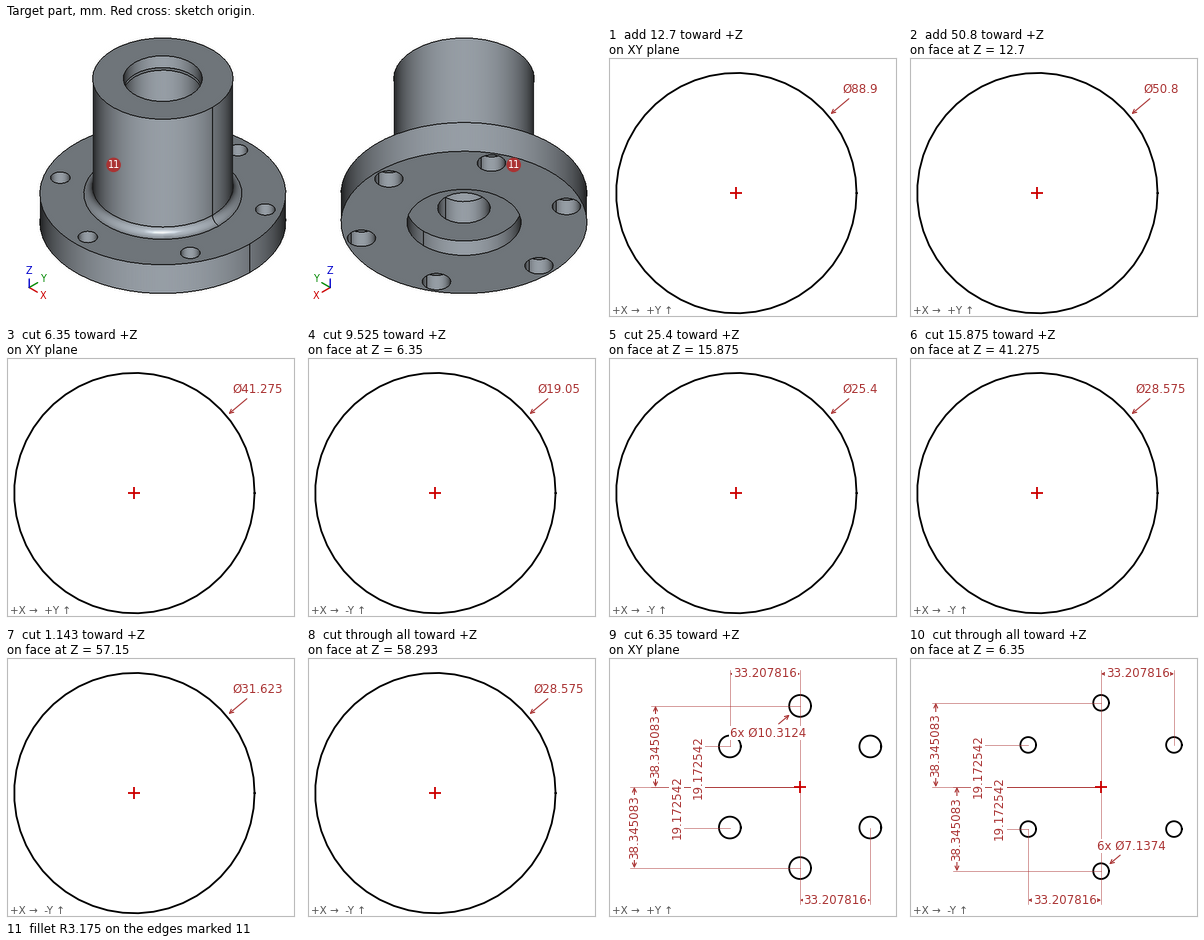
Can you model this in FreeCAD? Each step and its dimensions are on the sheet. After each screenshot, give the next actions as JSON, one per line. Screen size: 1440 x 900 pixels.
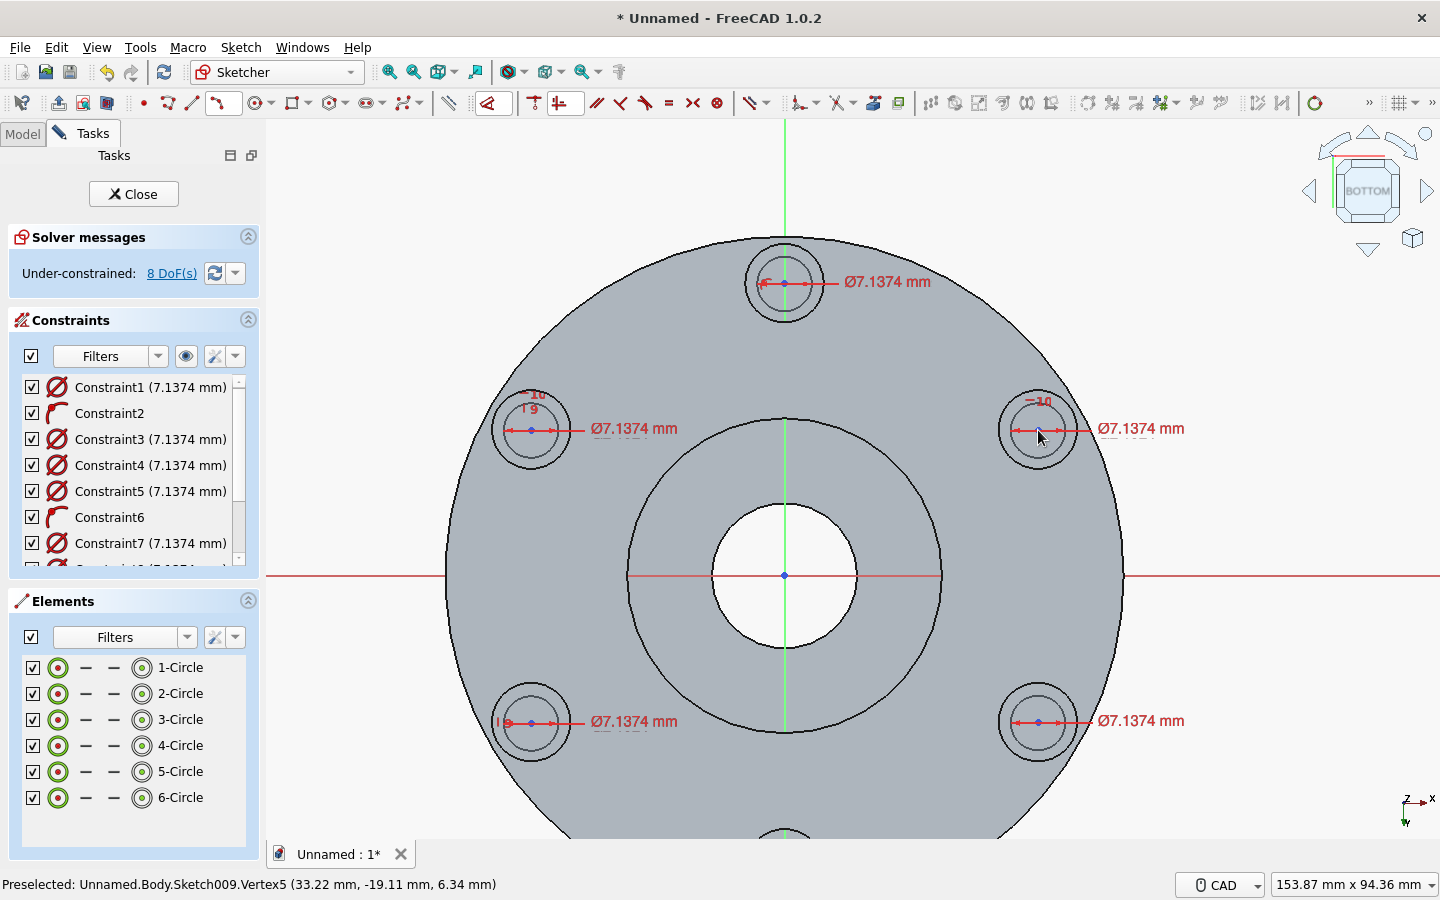
{"action": "left_click", "coordinate": [1038, 431]}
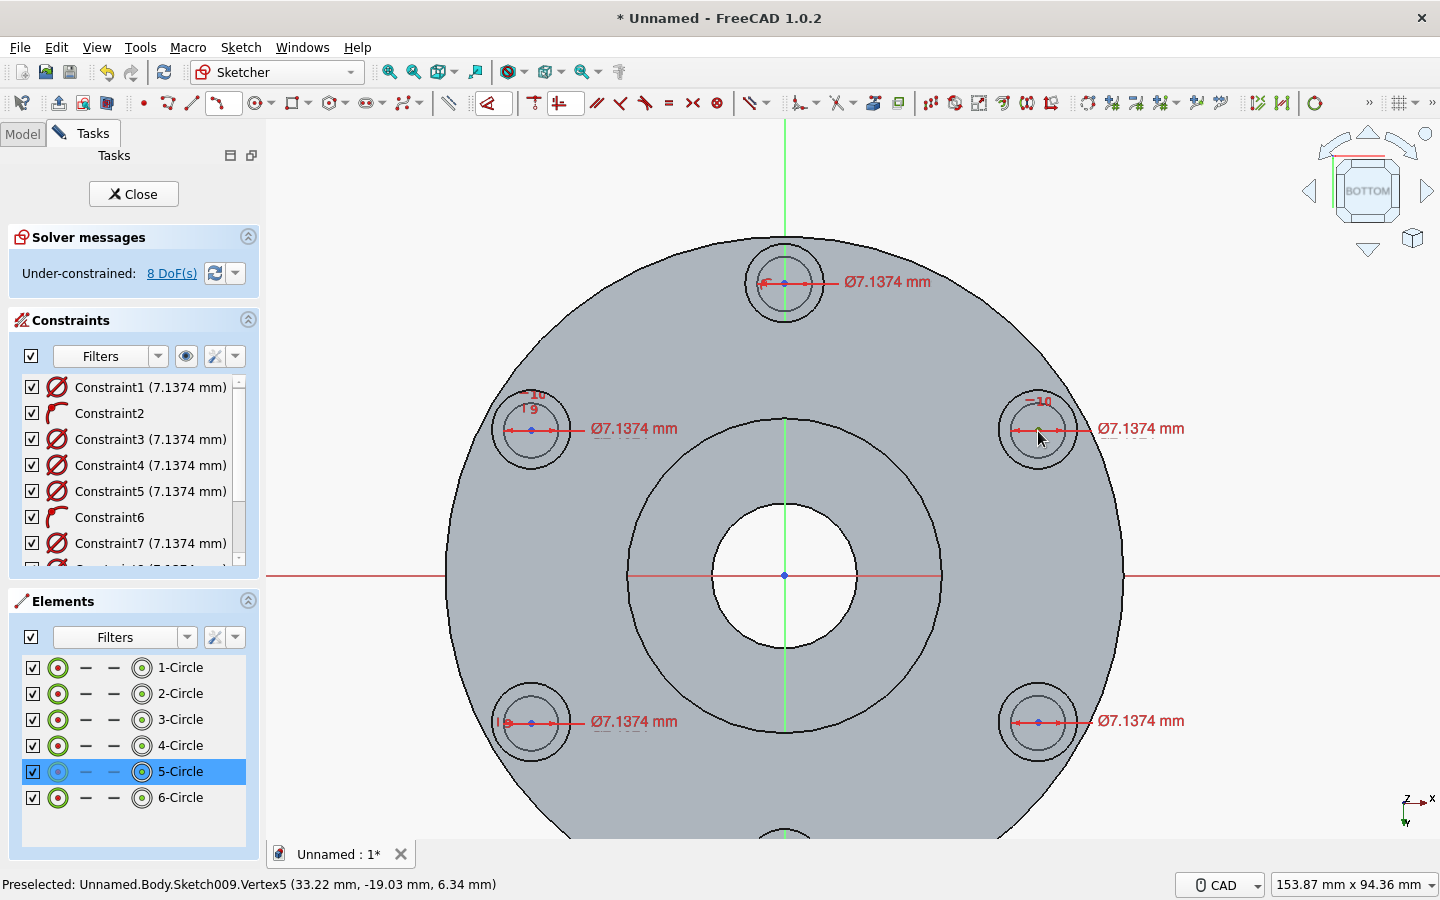
{"action": "left_click", "coordinate": [1038, 723]}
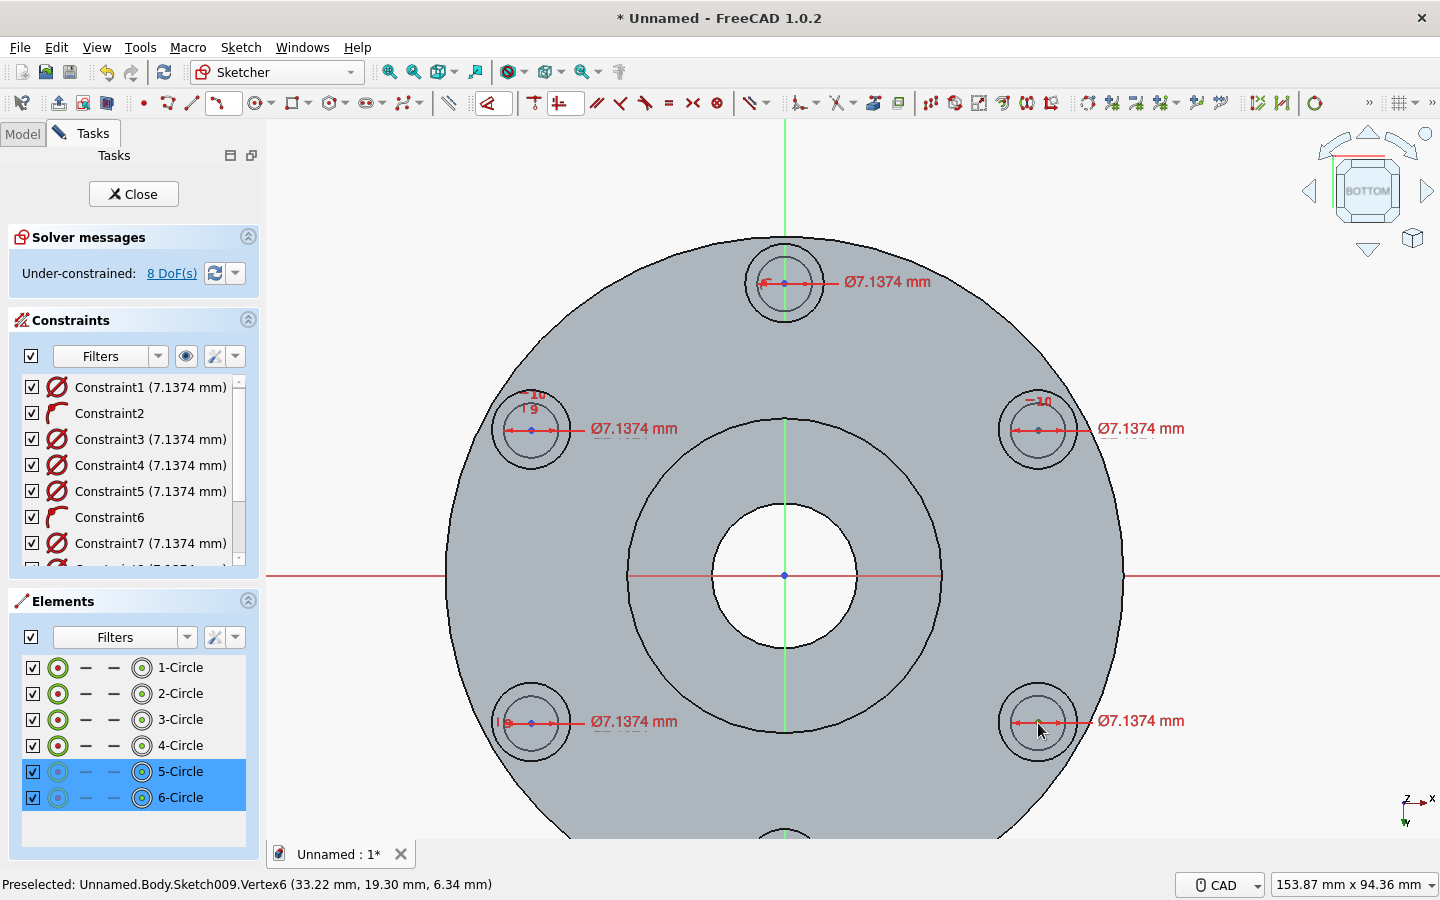
{"action": "key", "text": "v"}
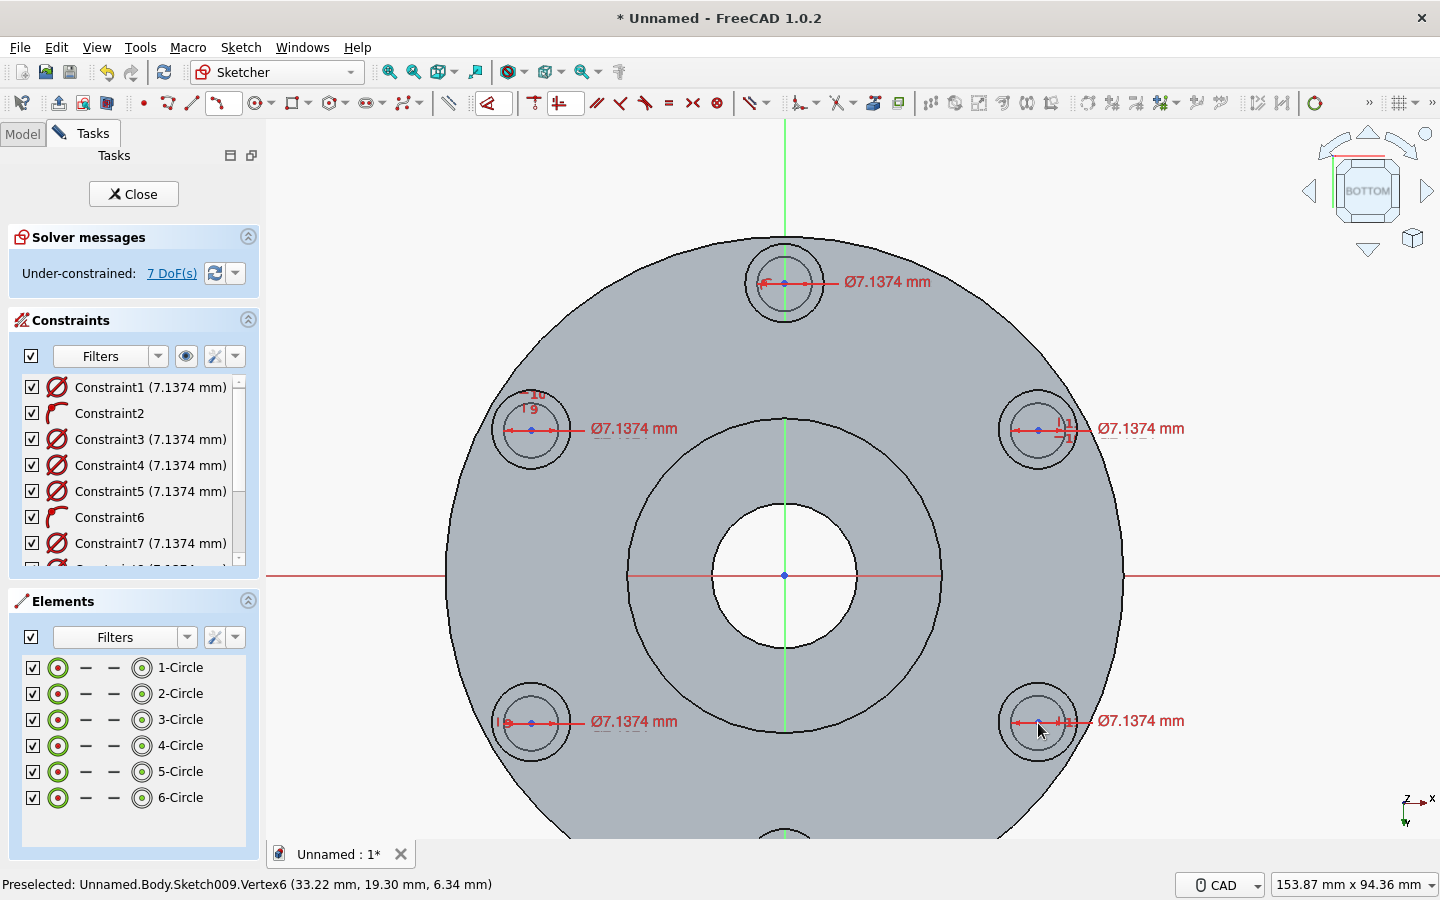
{"action": "left_click", "coordinate": [531, 724]}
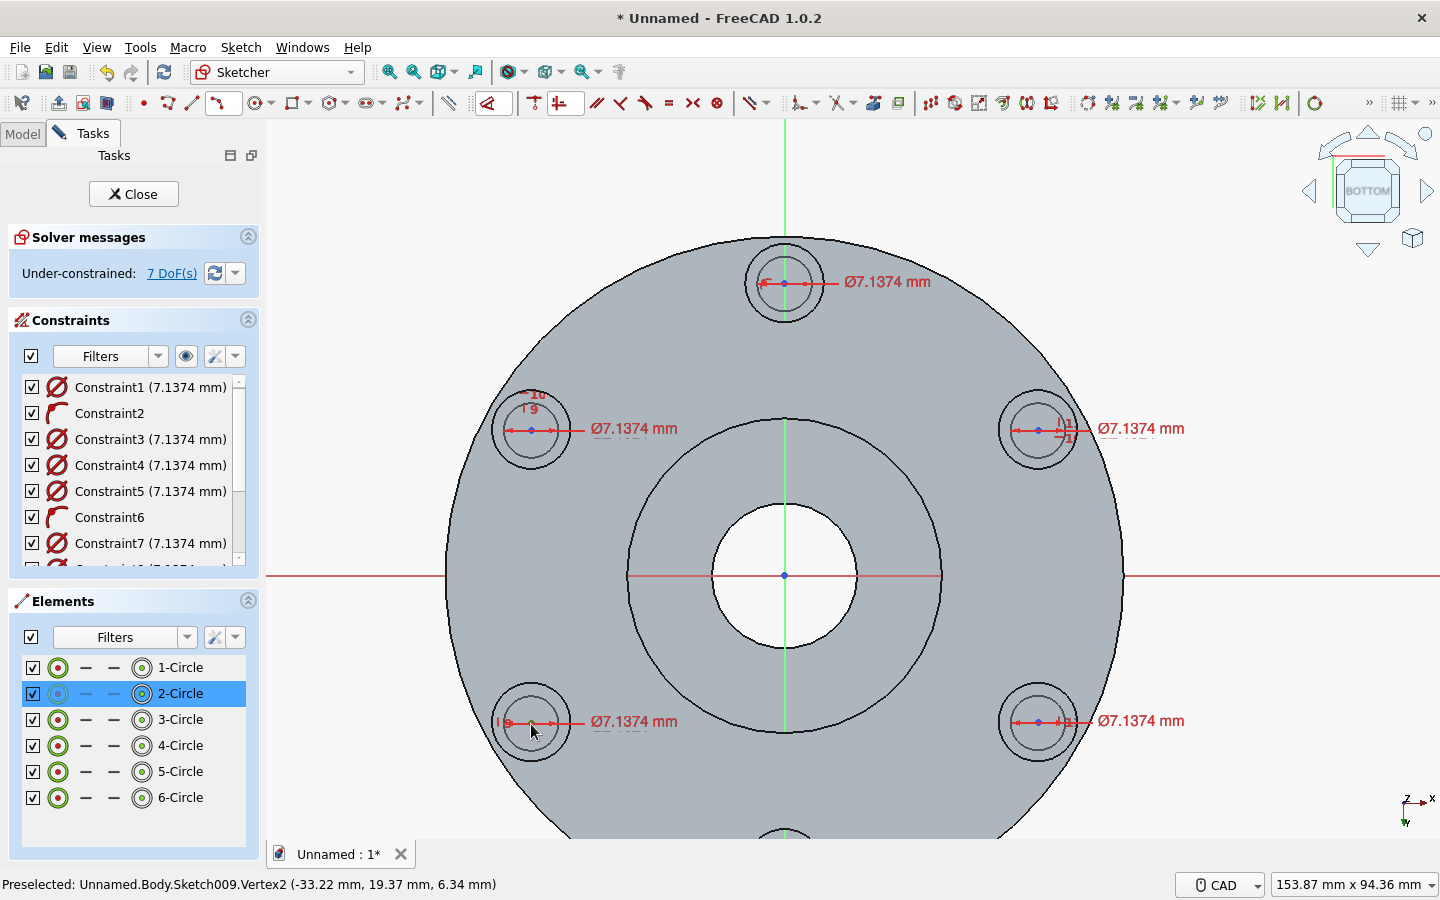
{"action": "left_click", "coordinate": [1038, 723]}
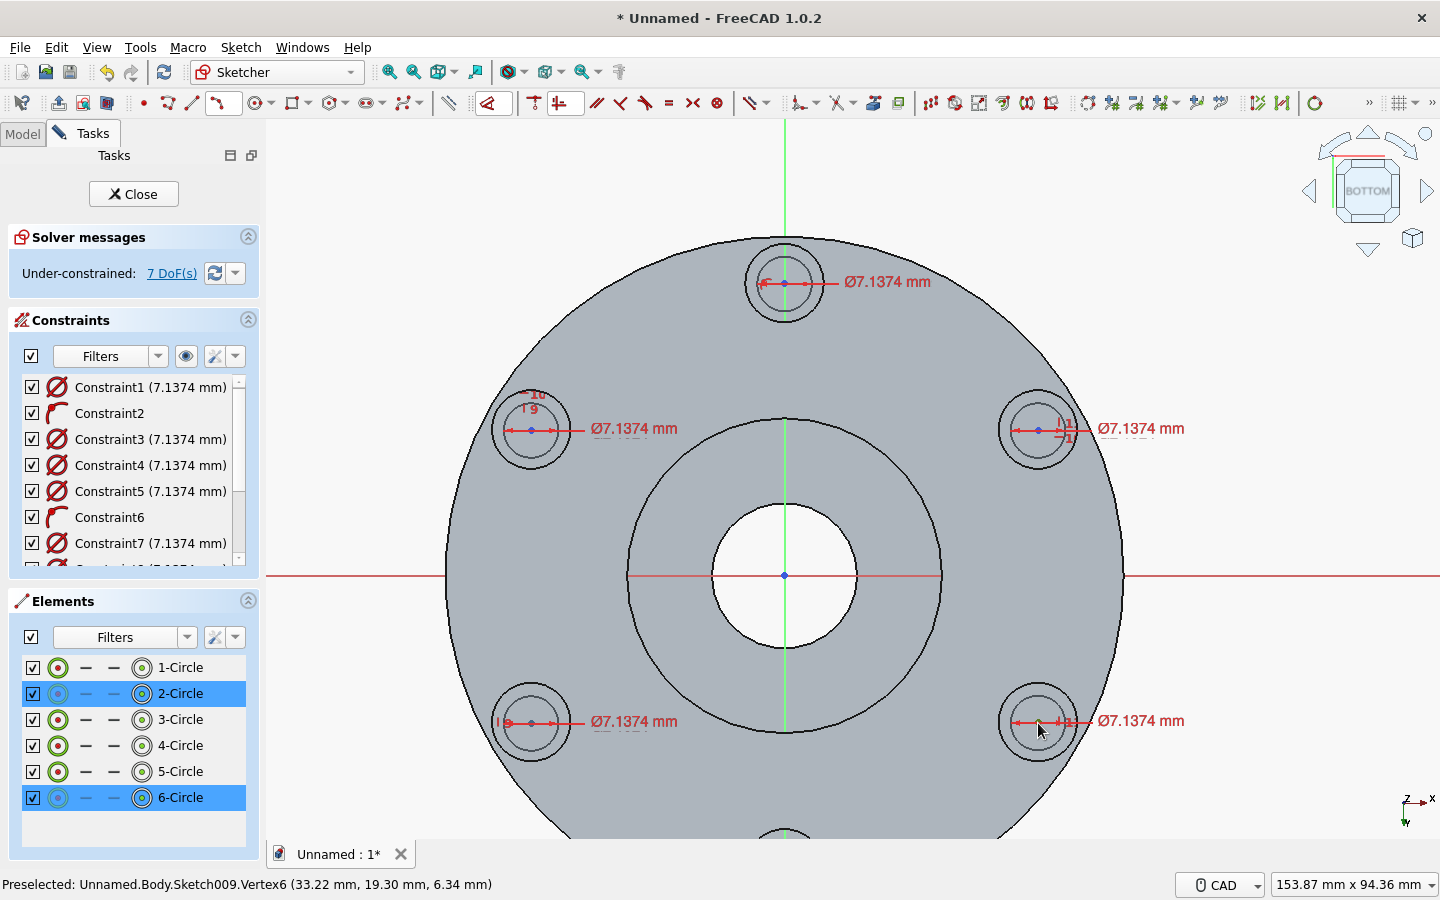
{"action": "key", "text": "h"}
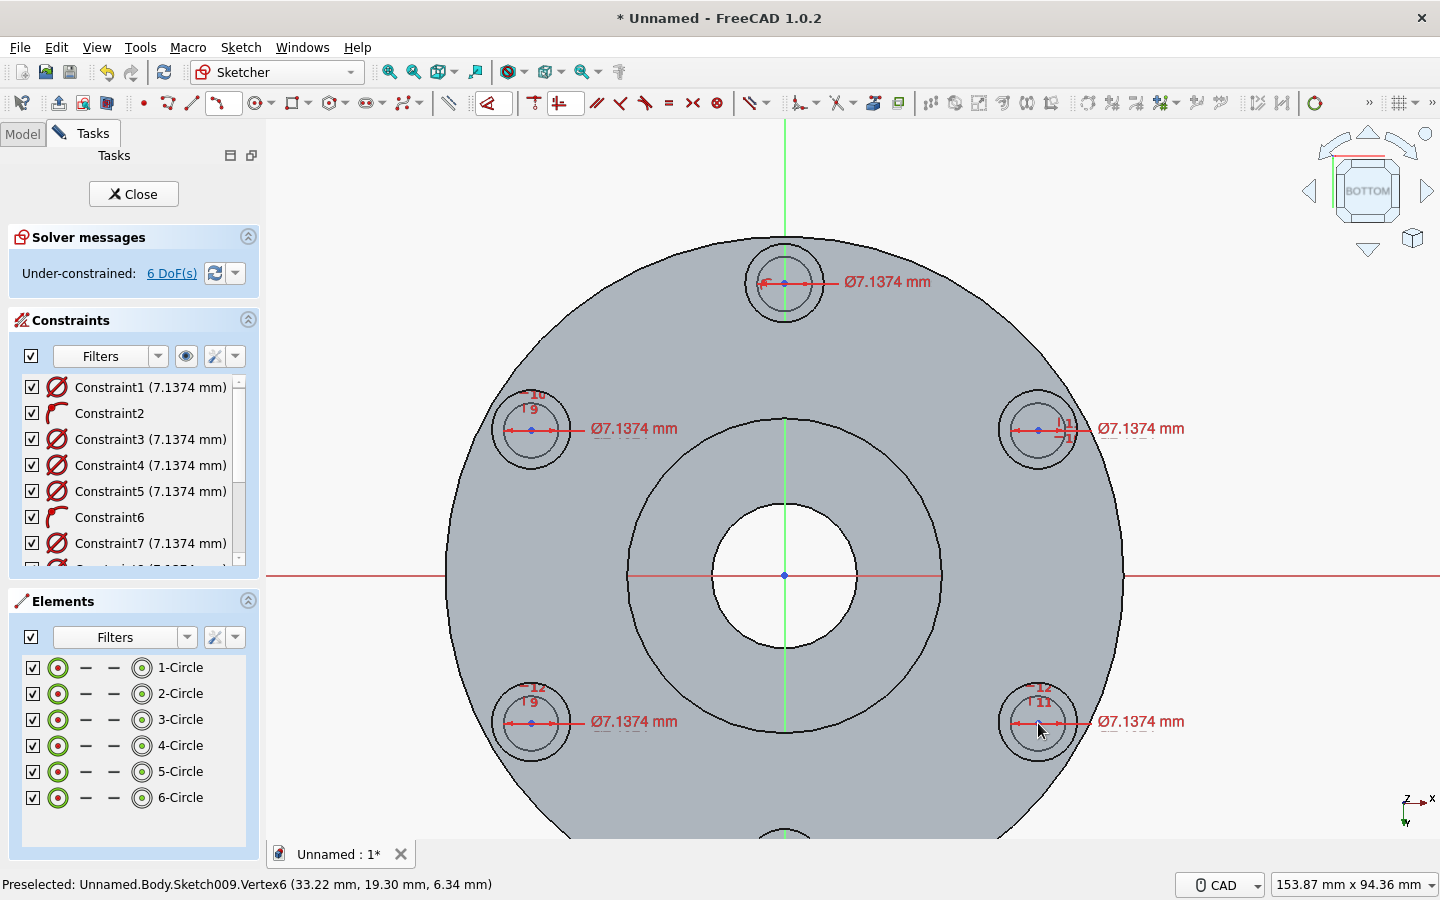
{"action": "key", "text": "d"}